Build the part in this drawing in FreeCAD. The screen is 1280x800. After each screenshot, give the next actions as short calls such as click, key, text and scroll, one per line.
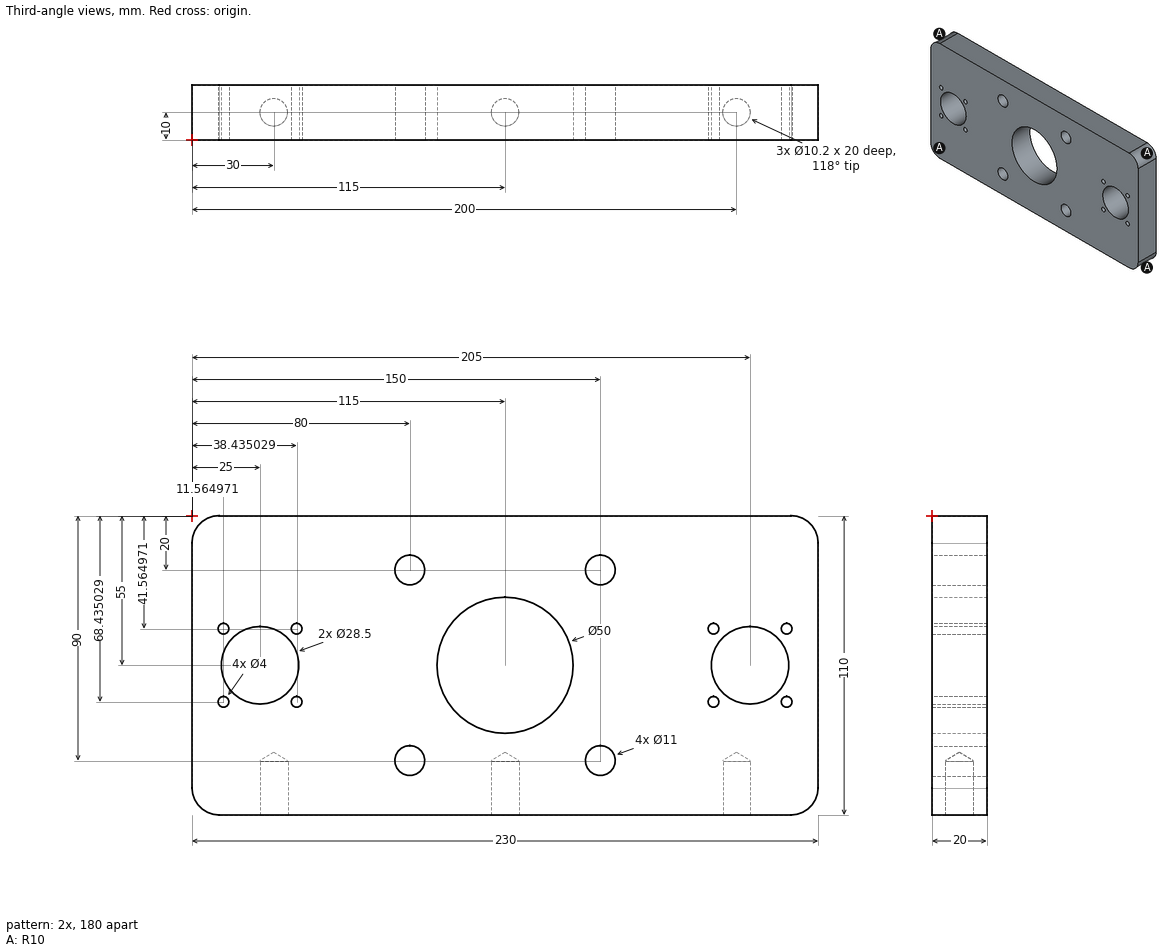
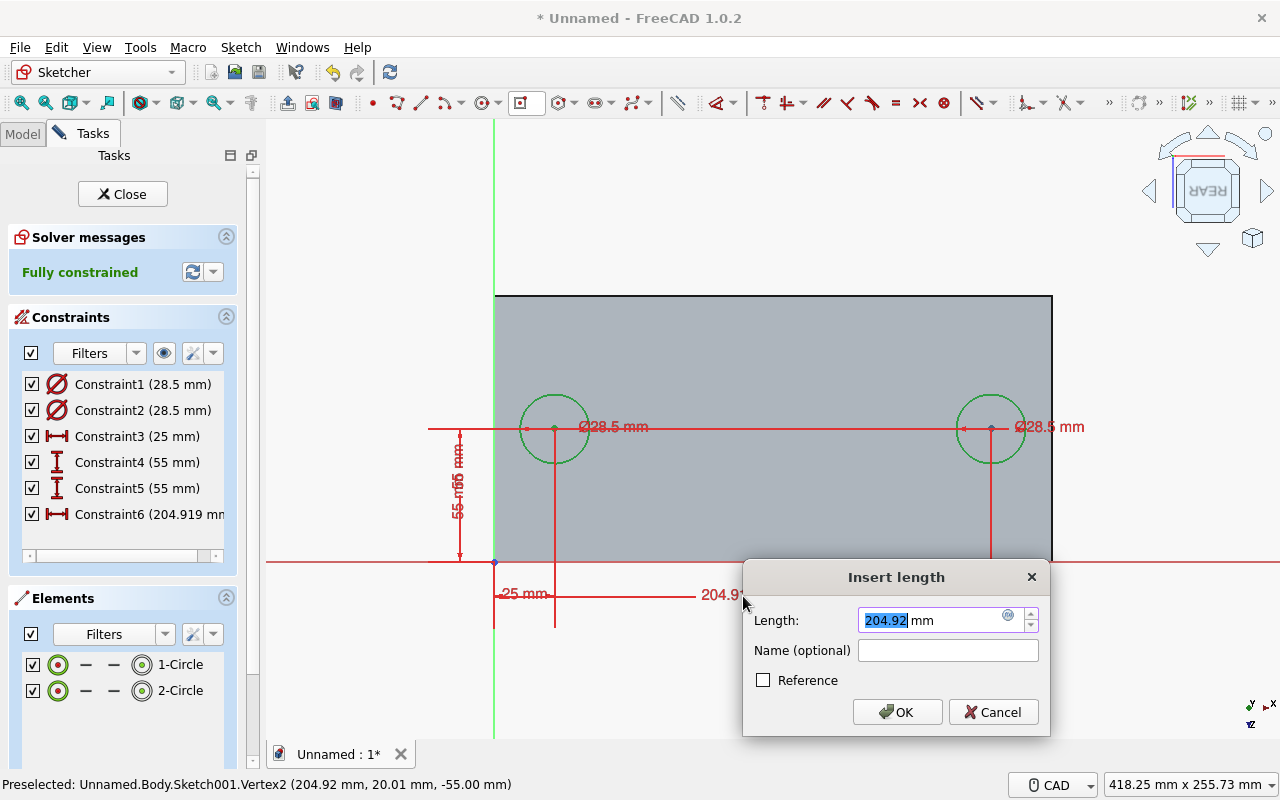
text(205)
key(Return)
key(Escape)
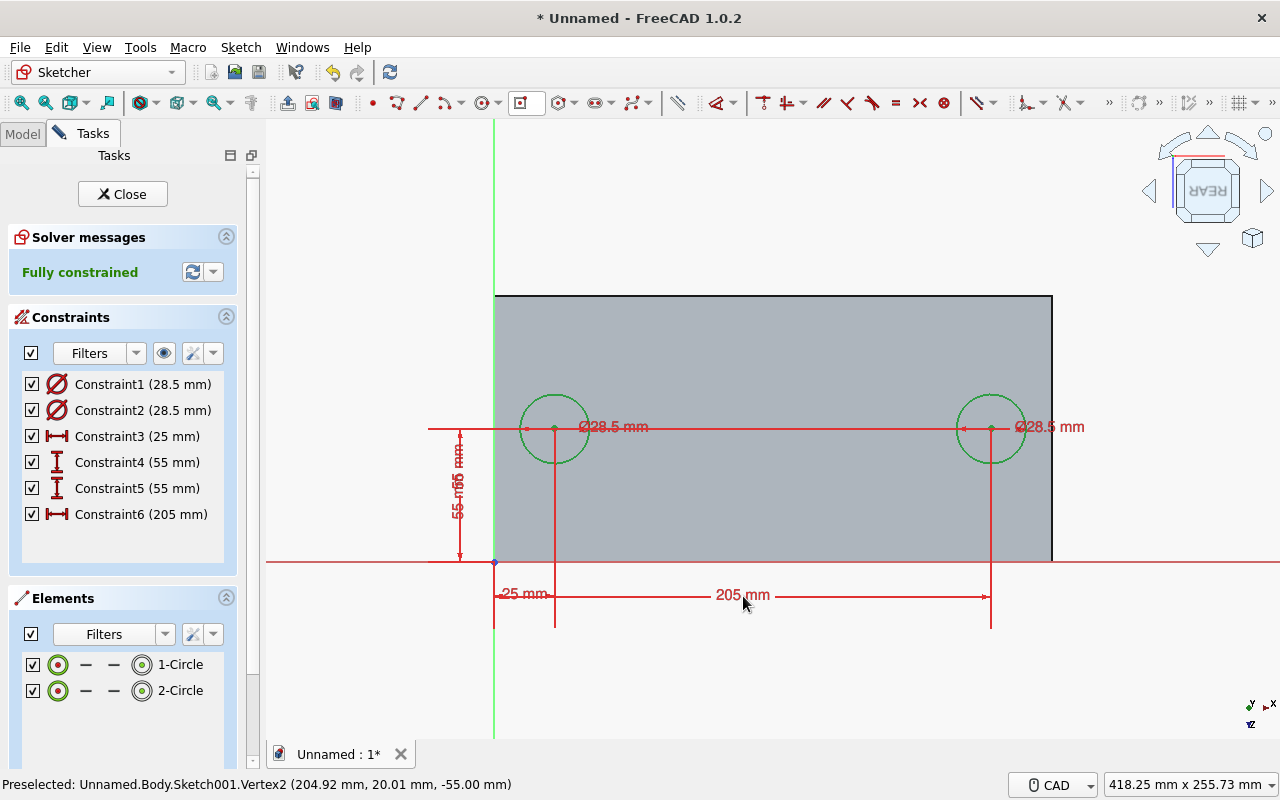
click(123, 194)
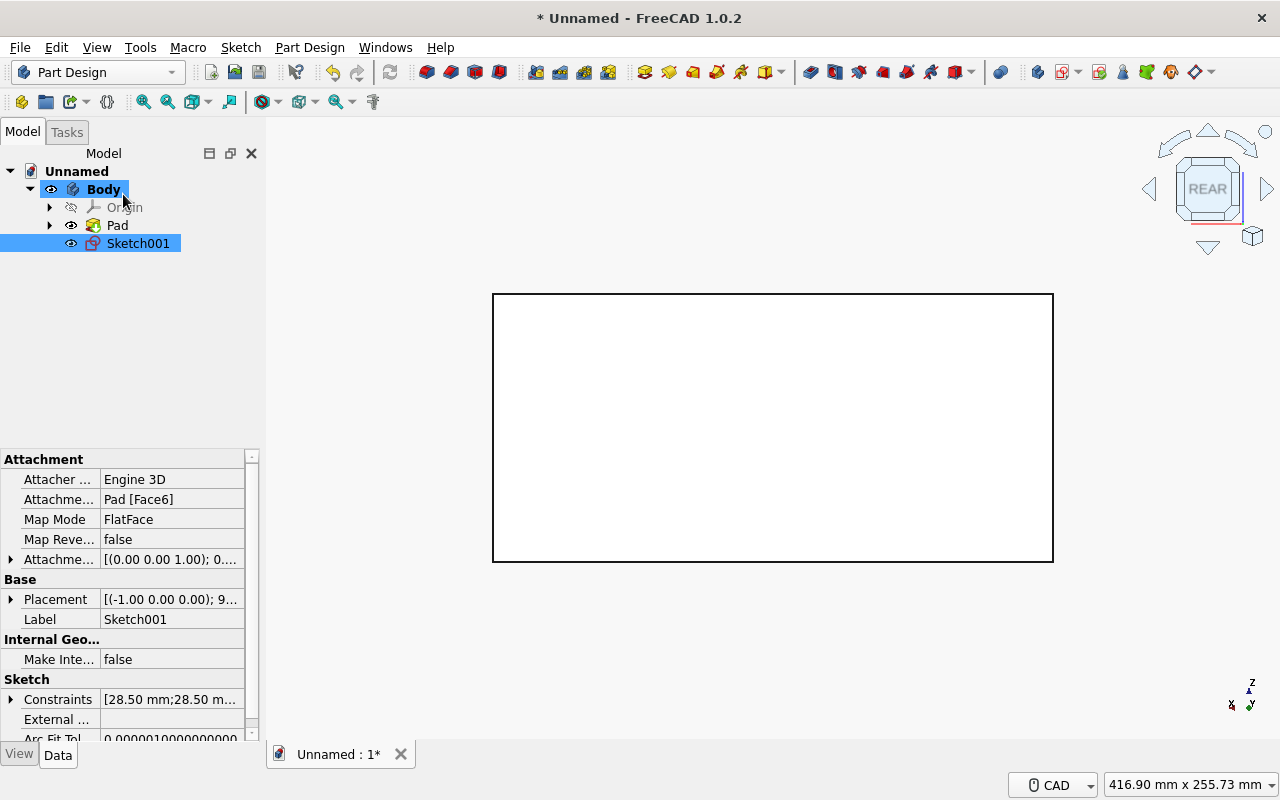
click(812, 72)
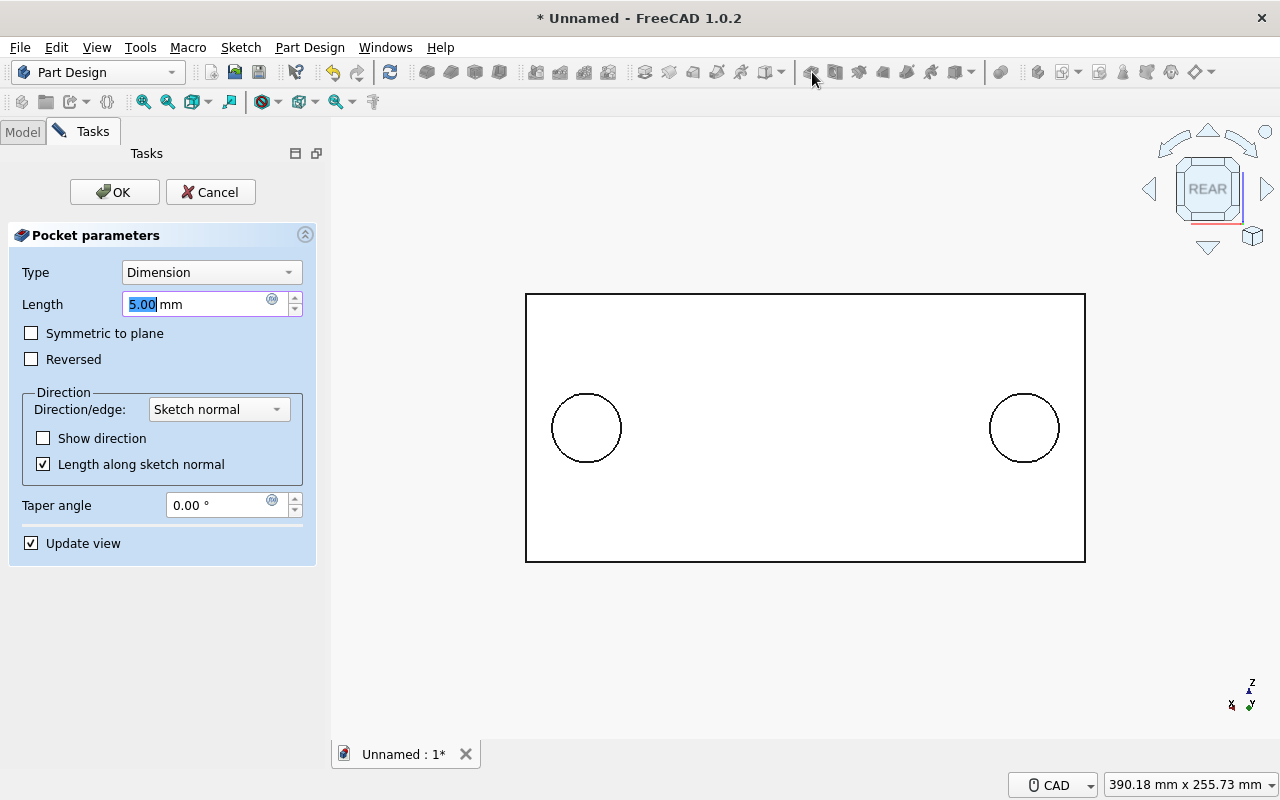
click(212, 272)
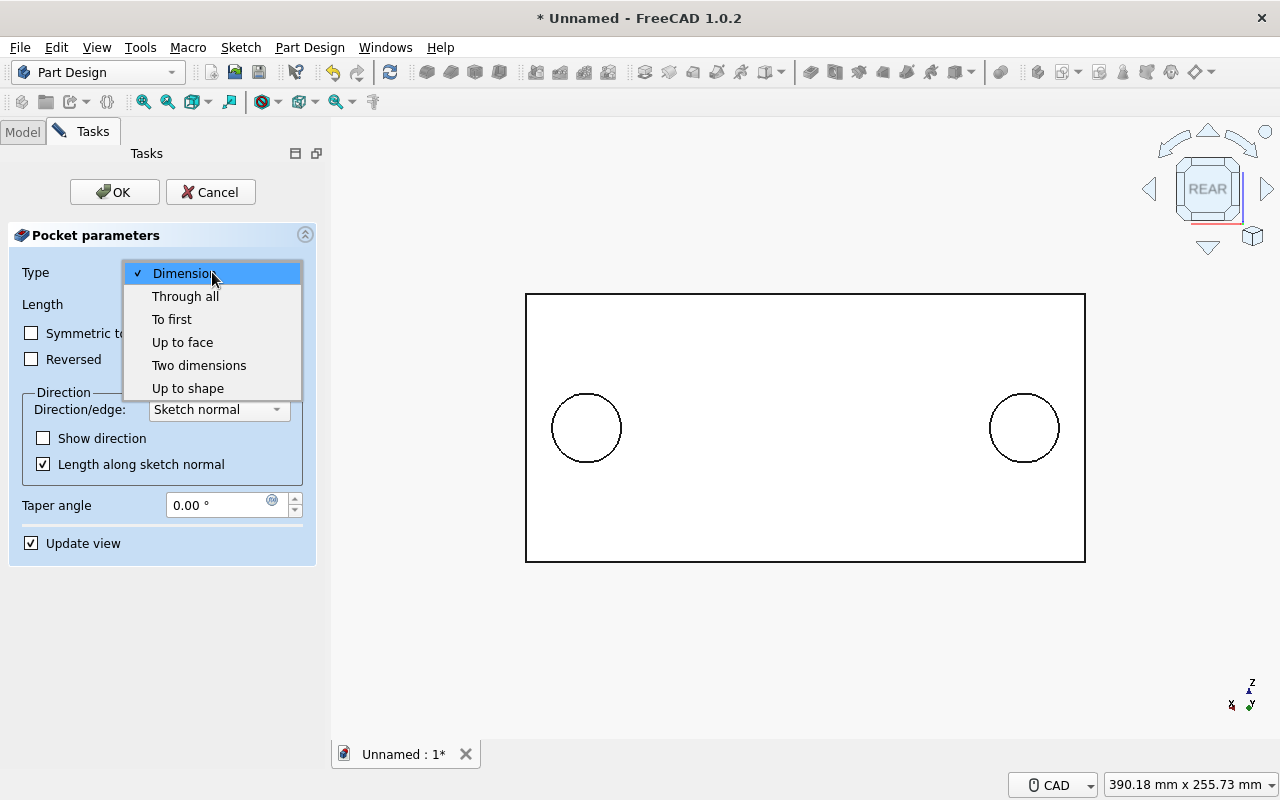
click(212, 296)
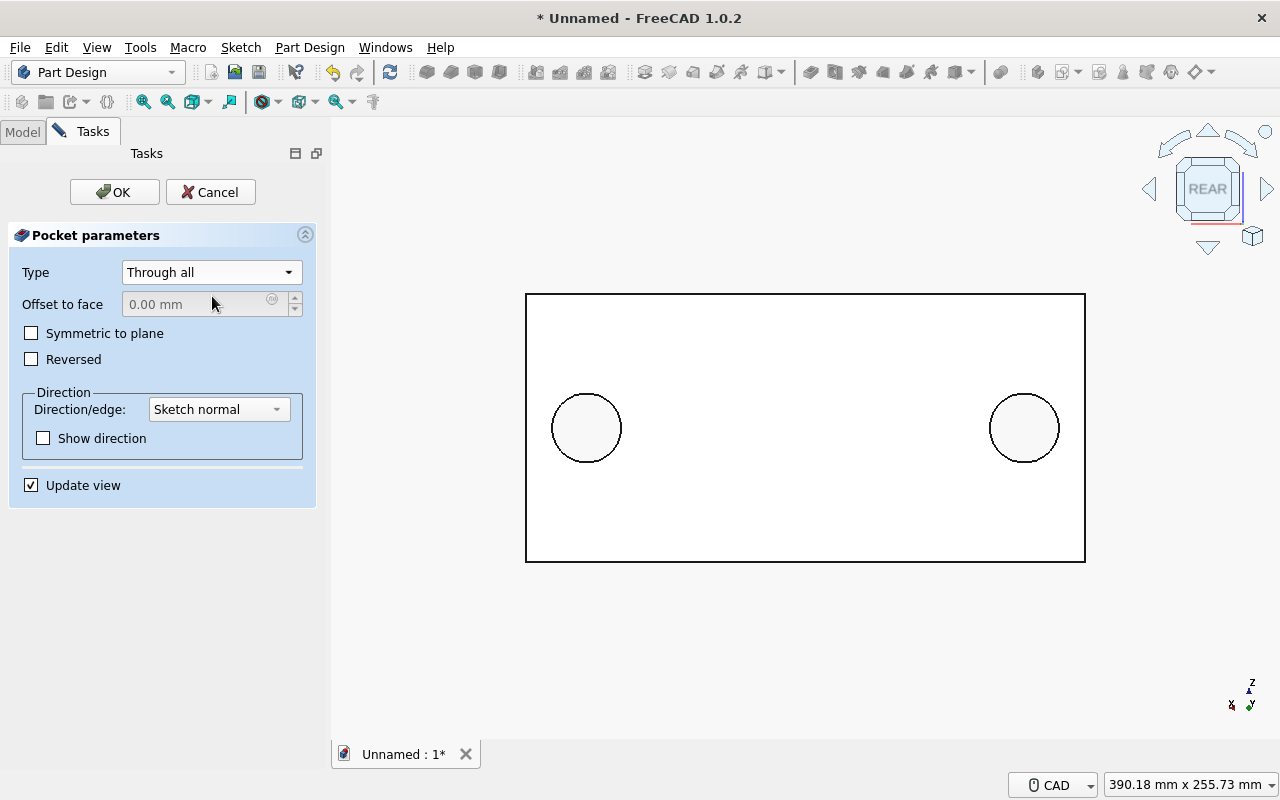
click(115, 192)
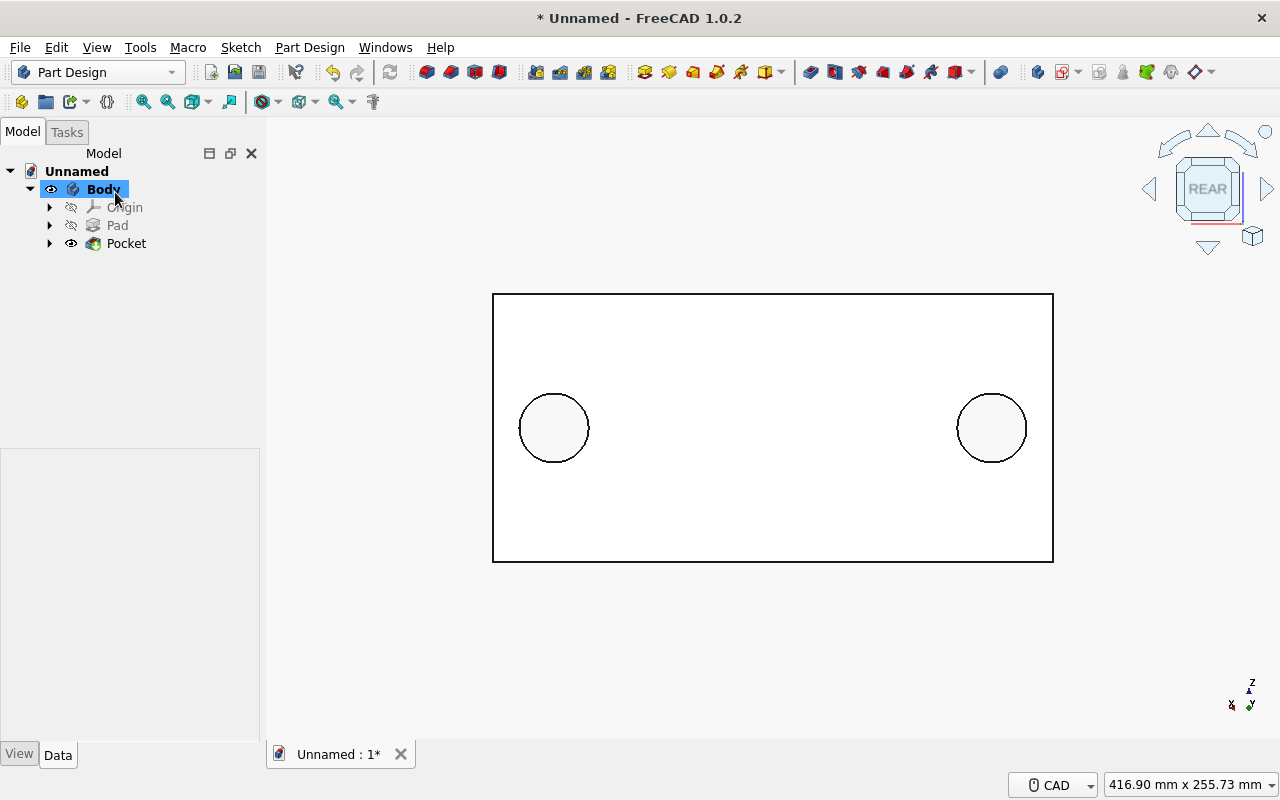
click(773, 427)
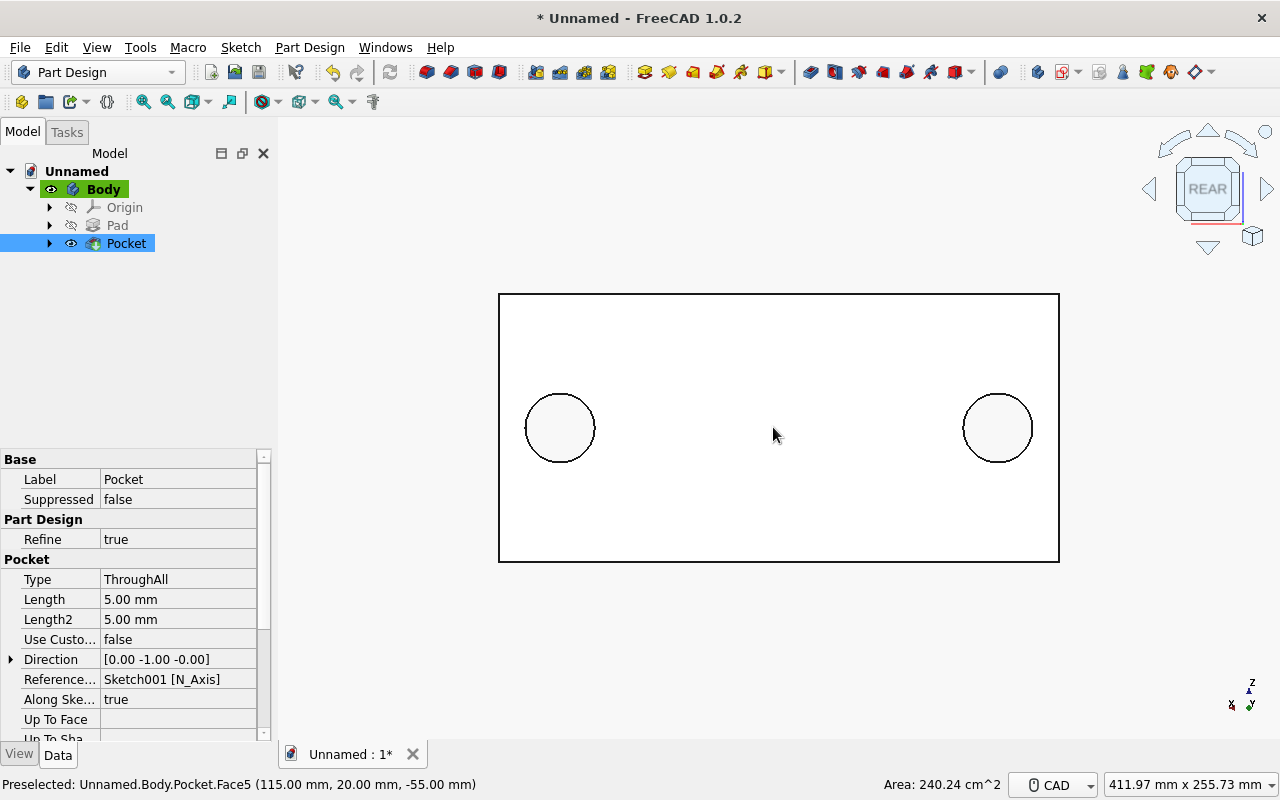
click(1062, 72)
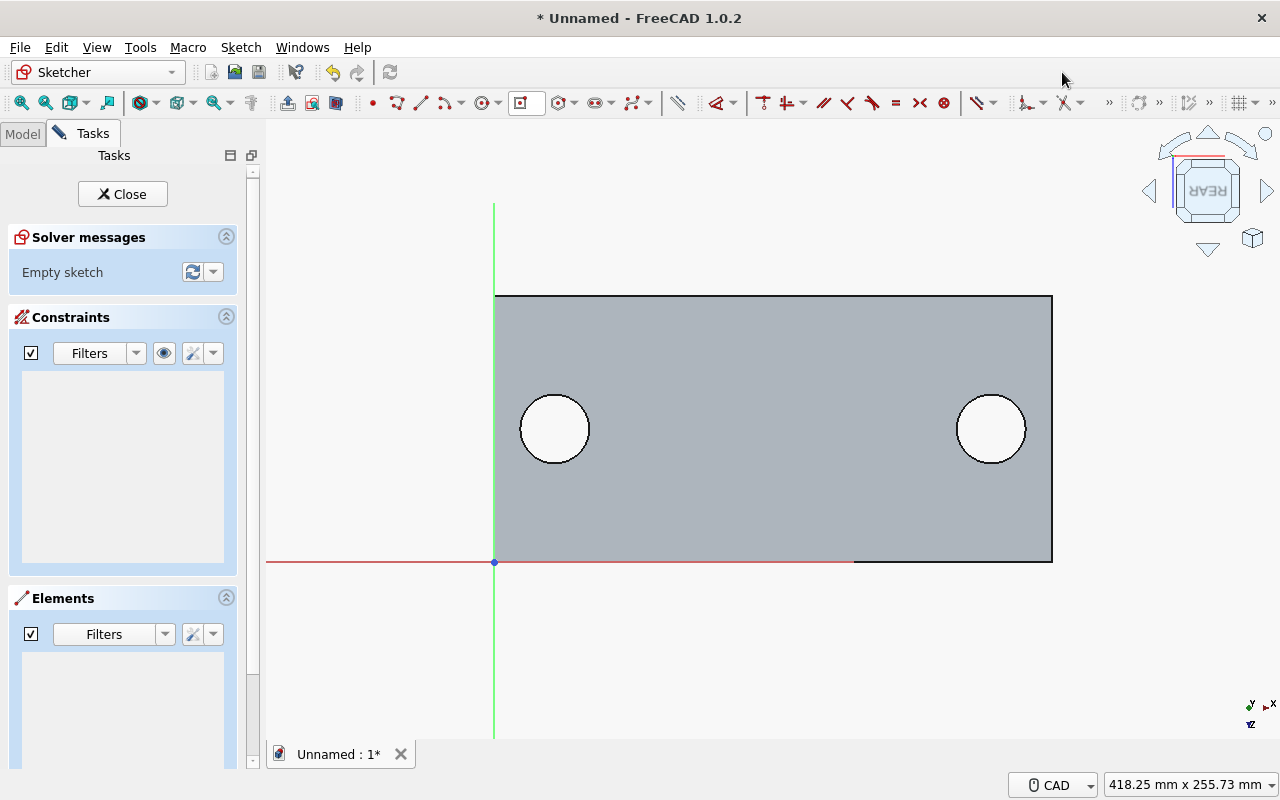
scroll(412, 516, up, 4)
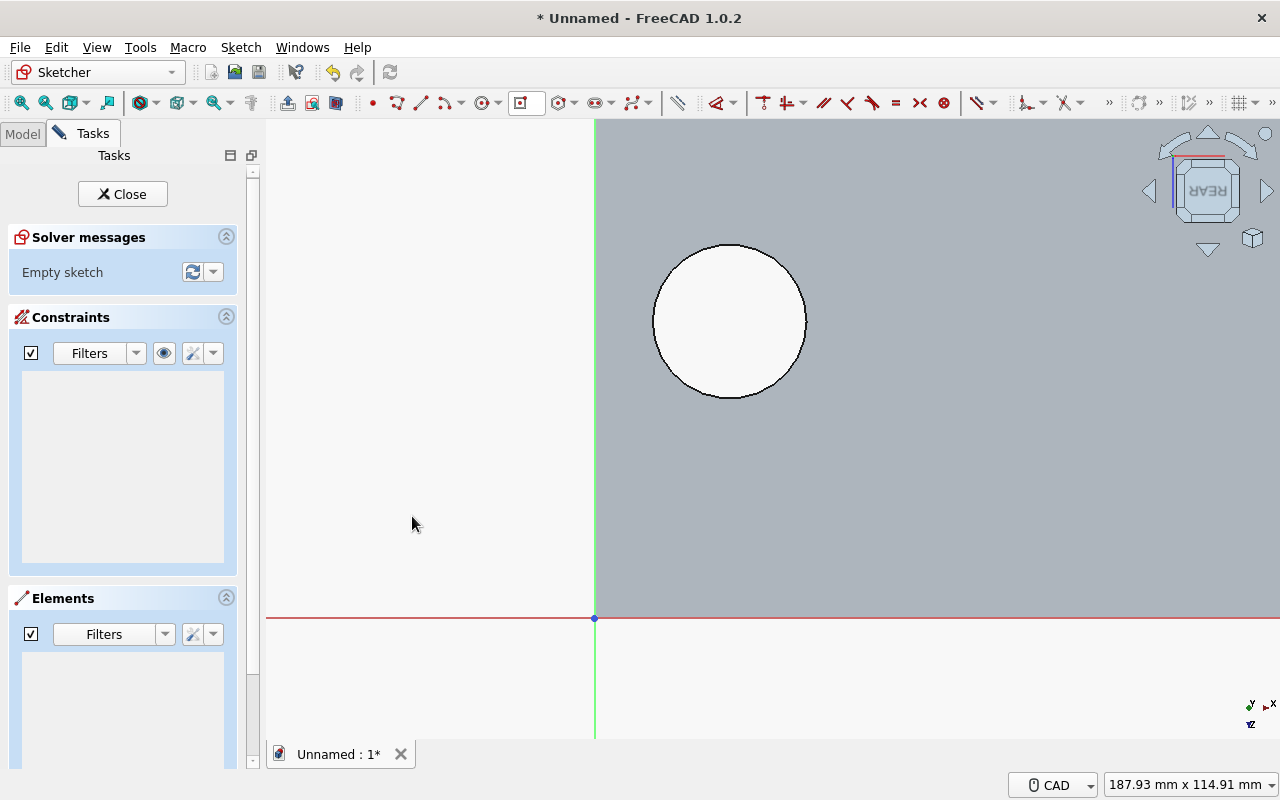
key(g)
key(c)